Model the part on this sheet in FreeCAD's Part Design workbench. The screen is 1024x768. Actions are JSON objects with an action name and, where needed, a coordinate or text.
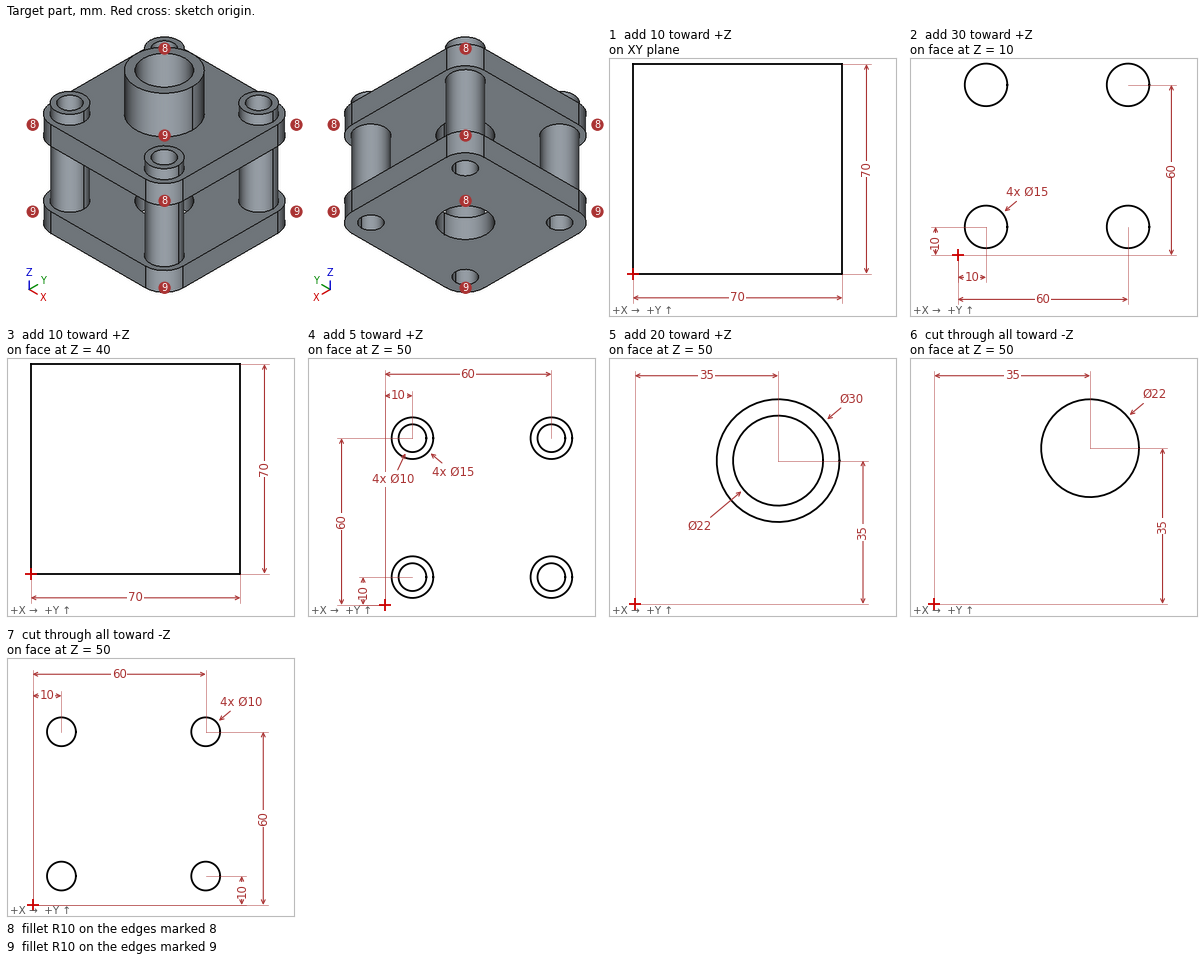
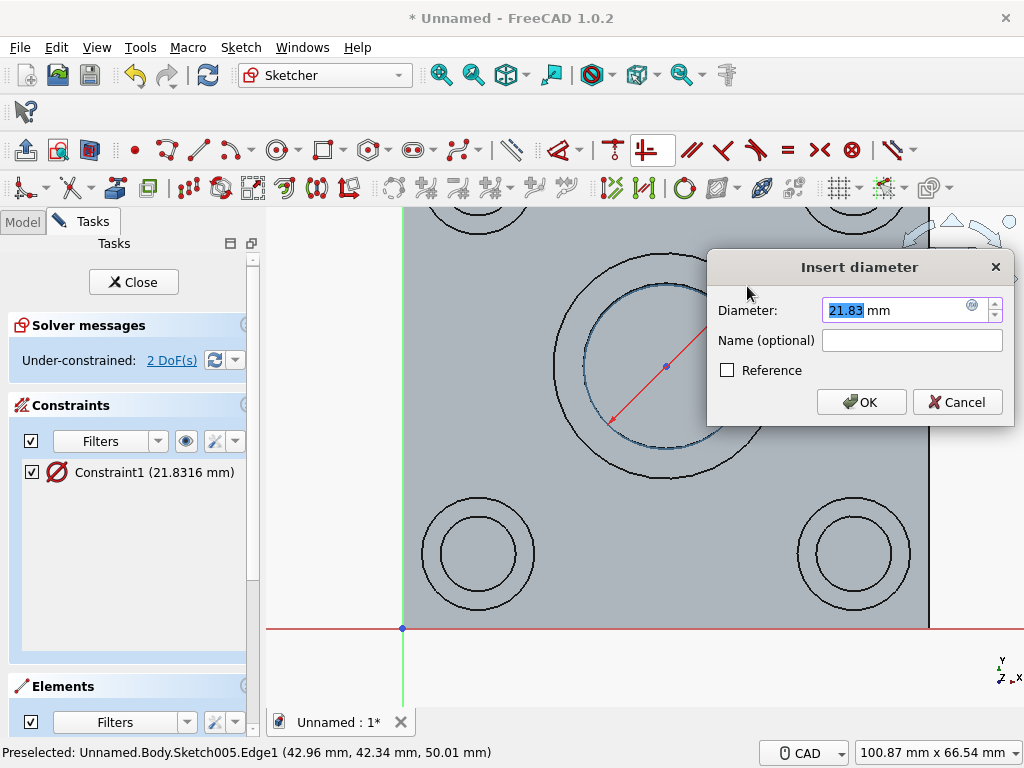
{"action": "type", "text": "22"}
{"action": "key", "text": "Return"}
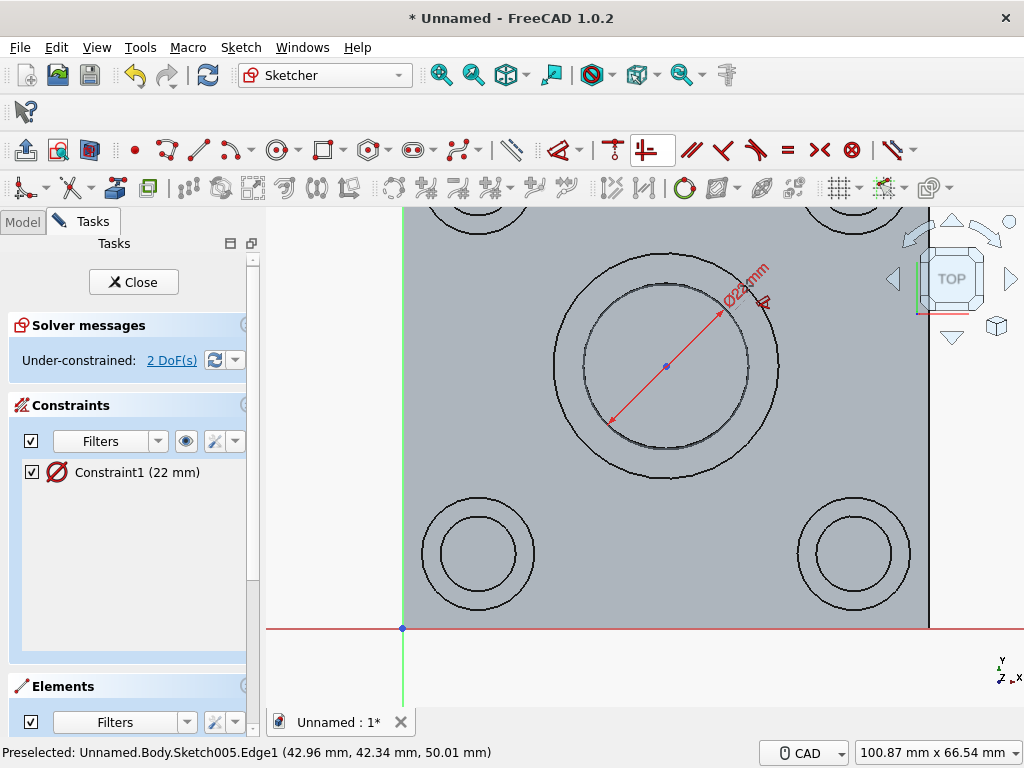
{"action": "left_click", "coordinate": [666, 367]}
{"action": "left_click", "coordinate": [534, 663]}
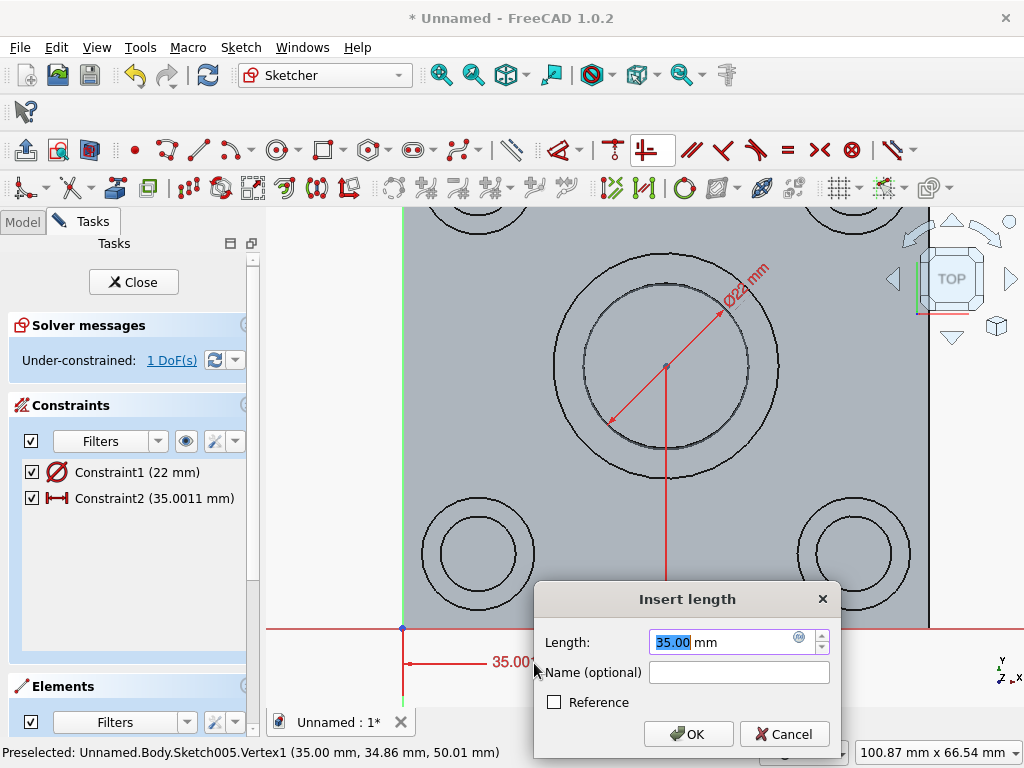
{"action": "type", "text": "35"}
{"action": "key", "text": "Return"}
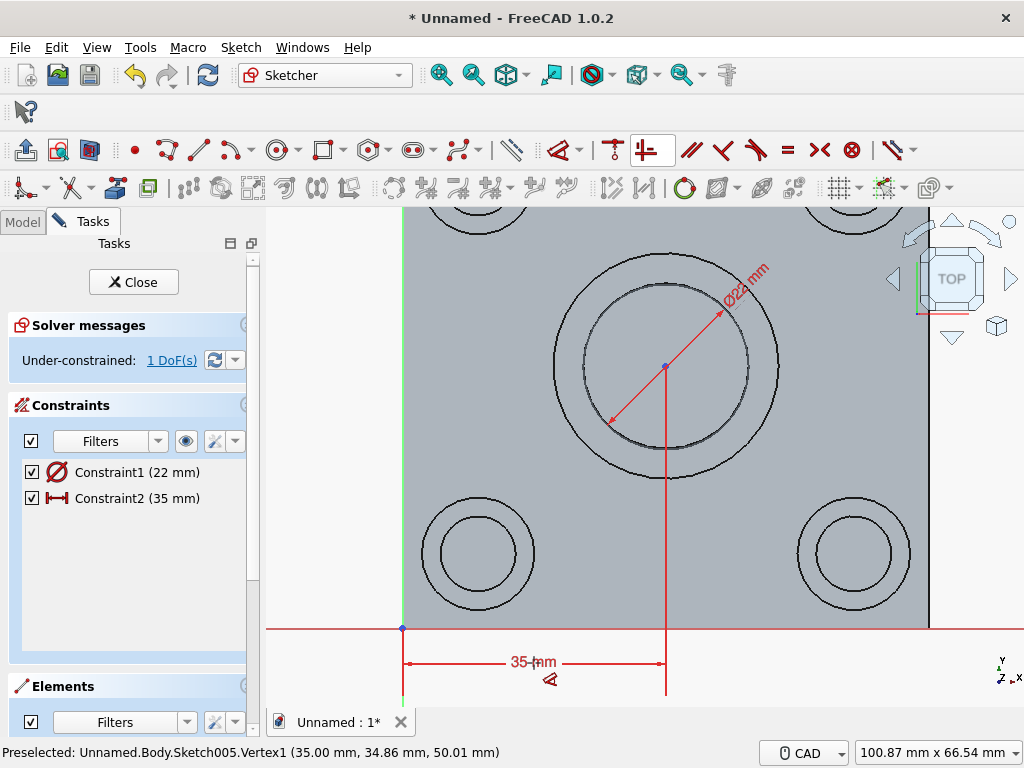
{"action": "left_click", "coordinate": [666, 367]}
{"action": "left_click", "coordinate": [369, 498]}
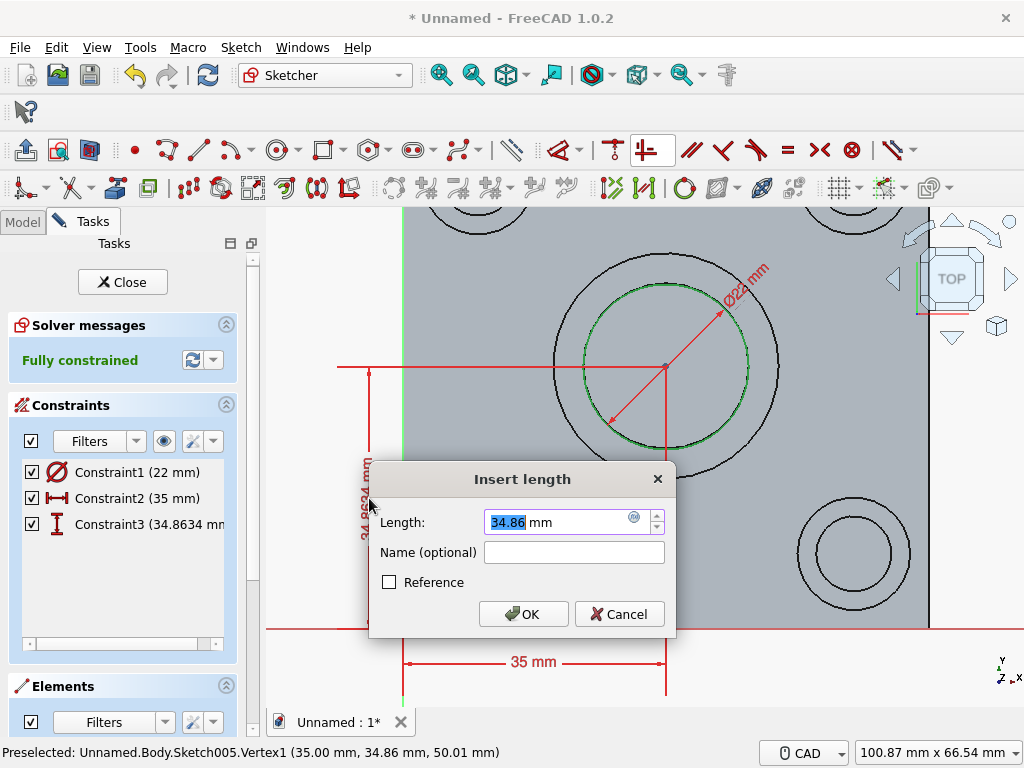
{"action": "type", "text": "35"}
{"action": "key", "text": "Return"}
{"action": "key", "text": "Escape"}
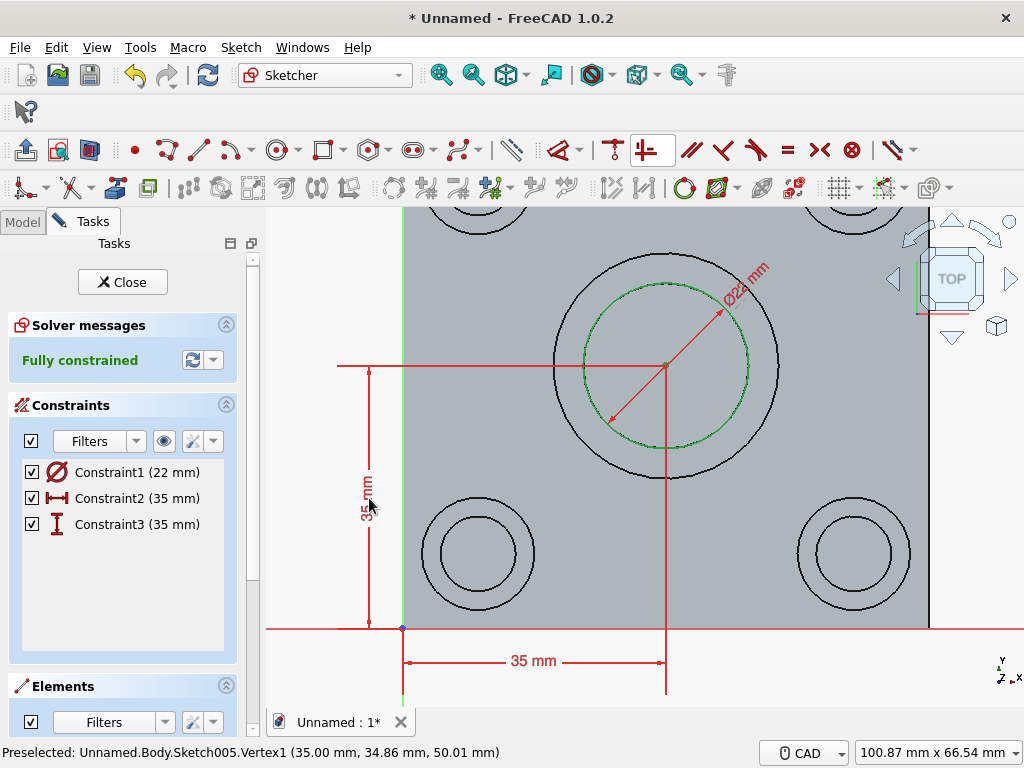
{"action": "left_click", "coordinate": [123, 282]}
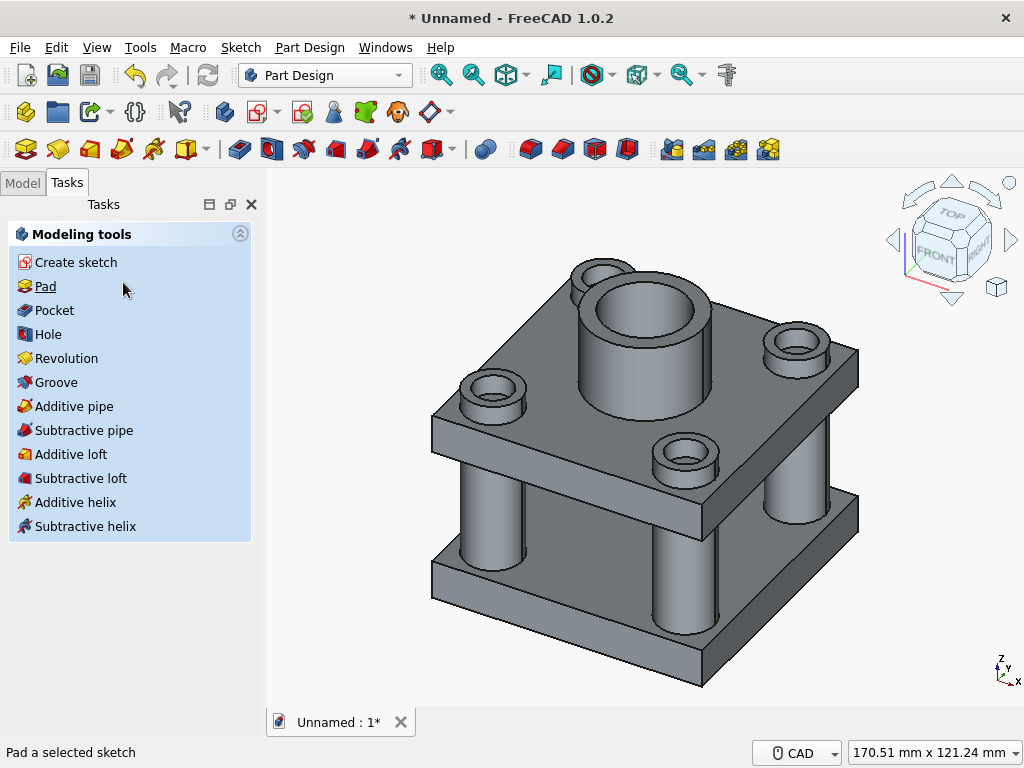
{"action": "left_click", "coordinate": [240, 150]}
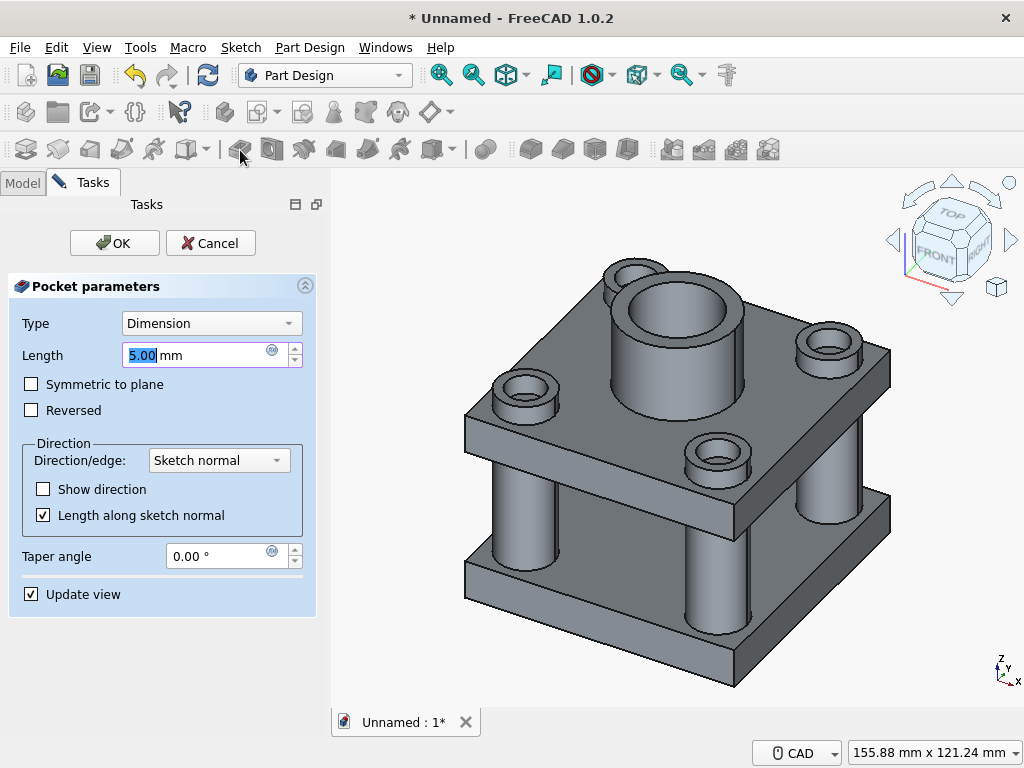
{"action": "left_click", "coordinate": [212, 324]}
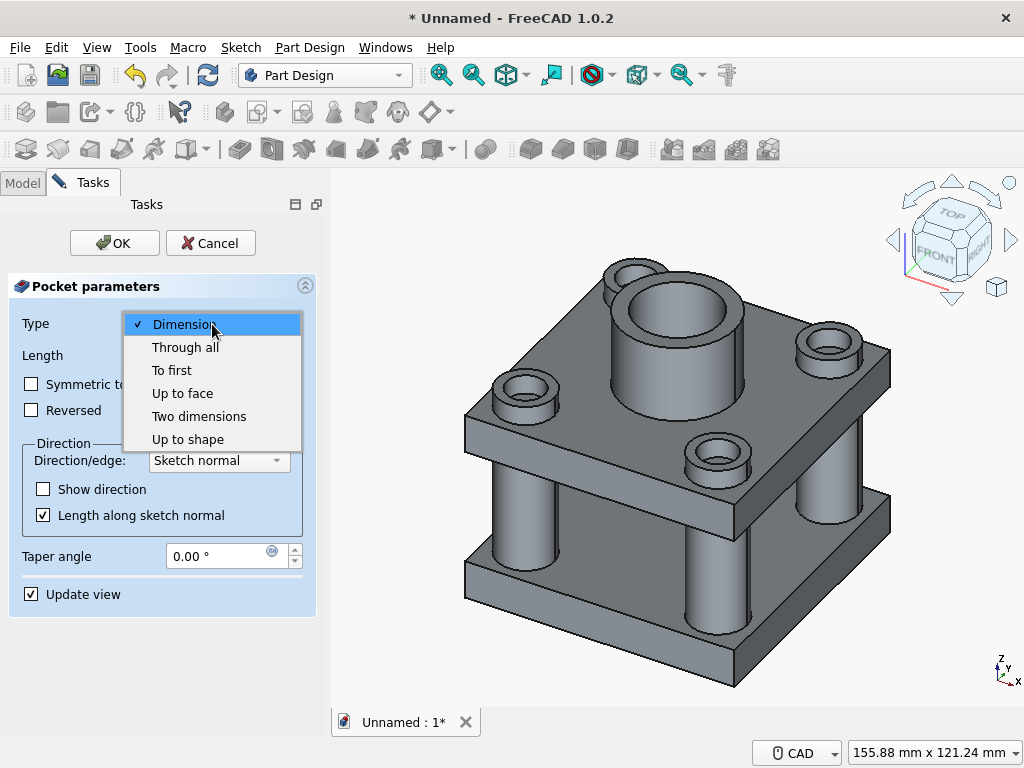
{"action": "left_click", "coordinate": [212, 348]}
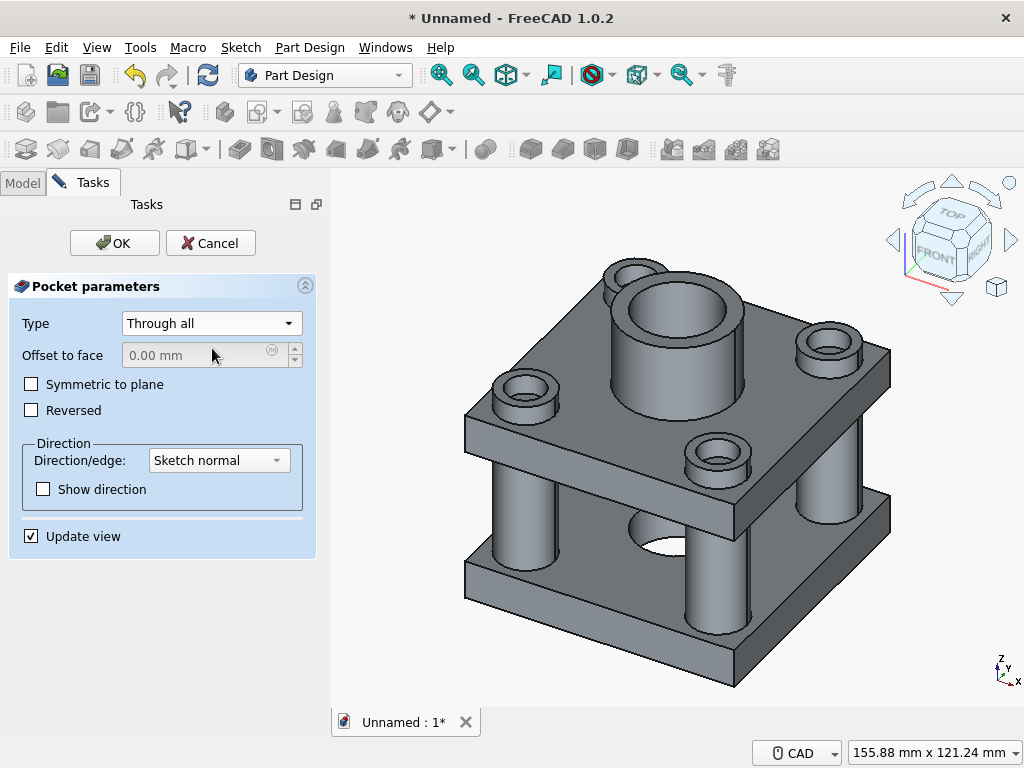
{"action": "left_click", "coordinate": [115, 243]}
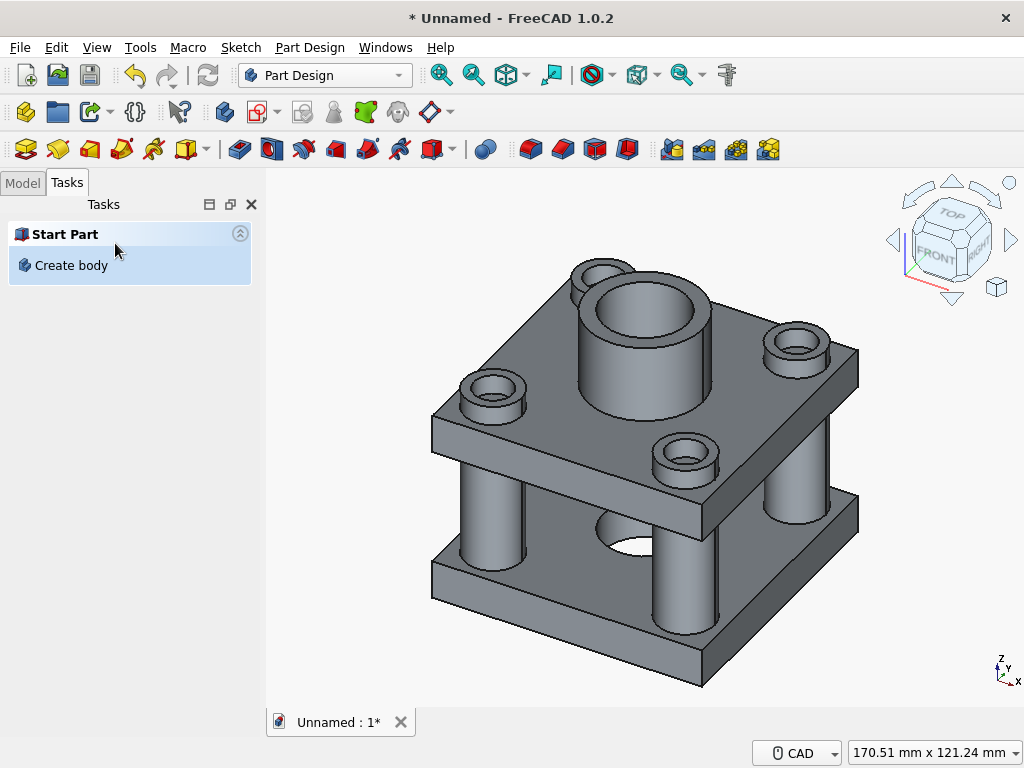
{"action": "left_click", "coordinate": [744, 385]}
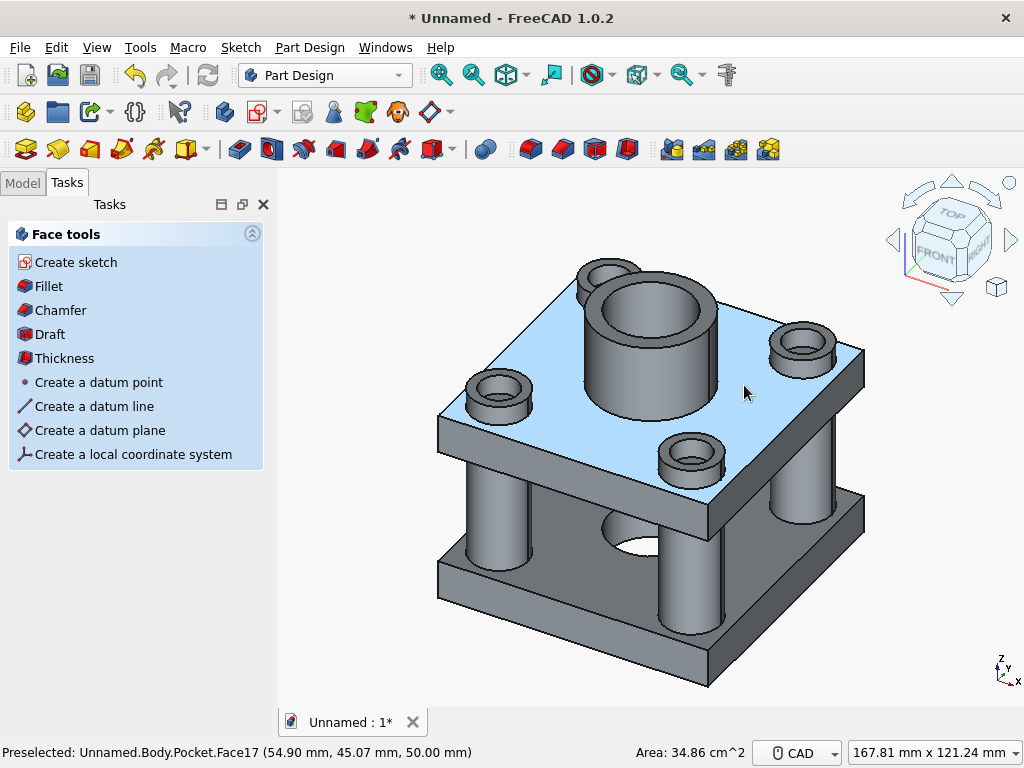
{"action": "left_click", "coordinate": [258, 112]}